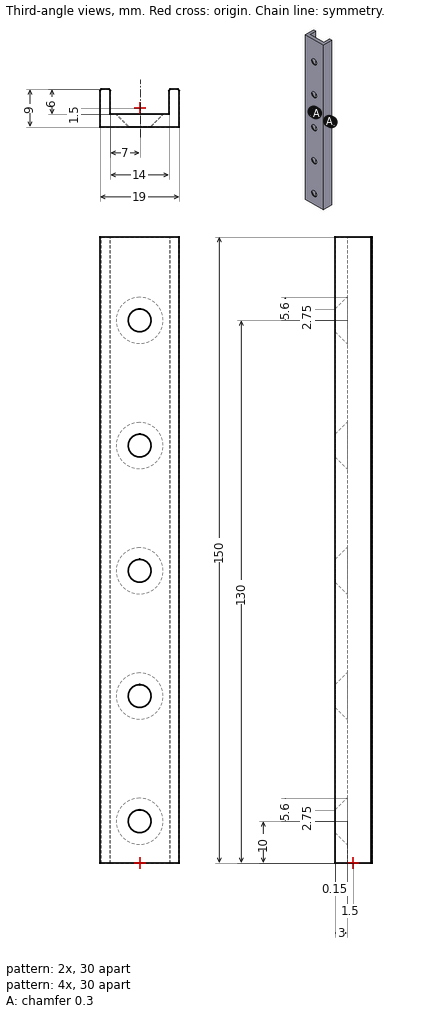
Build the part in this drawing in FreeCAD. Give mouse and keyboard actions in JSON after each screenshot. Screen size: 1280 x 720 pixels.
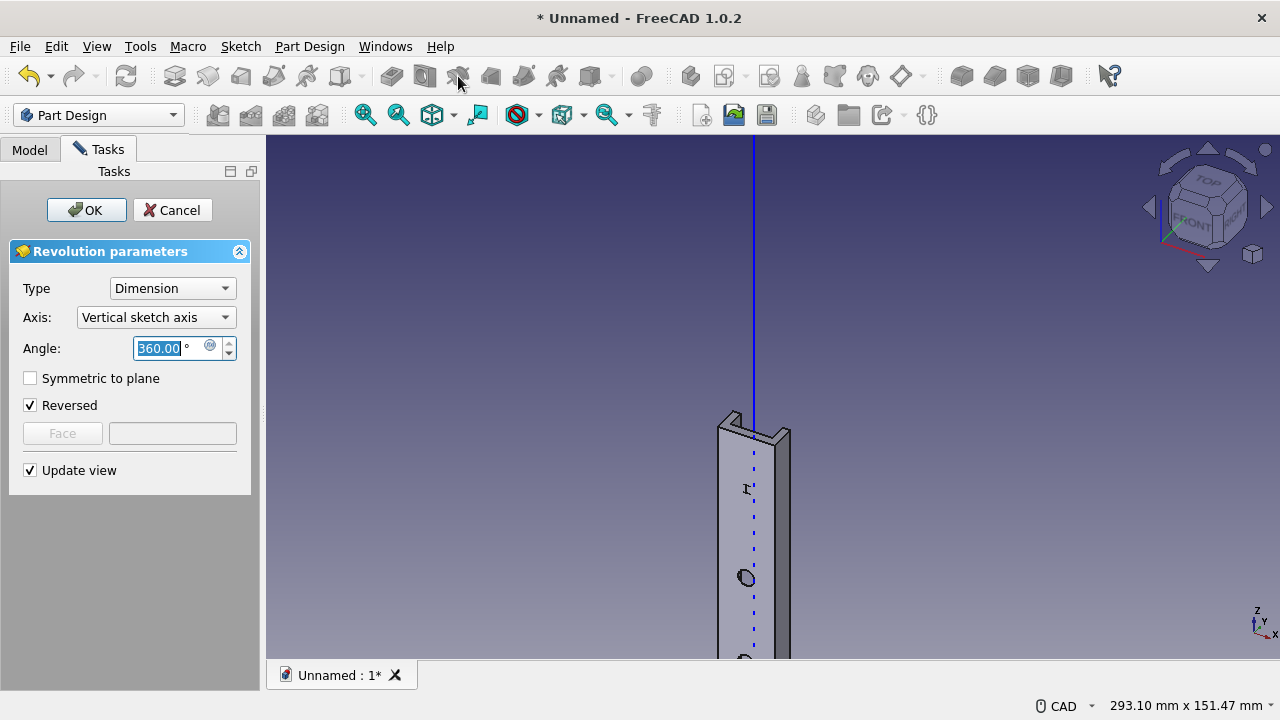
{"action": "left_click", "coordinate": [157, 318]}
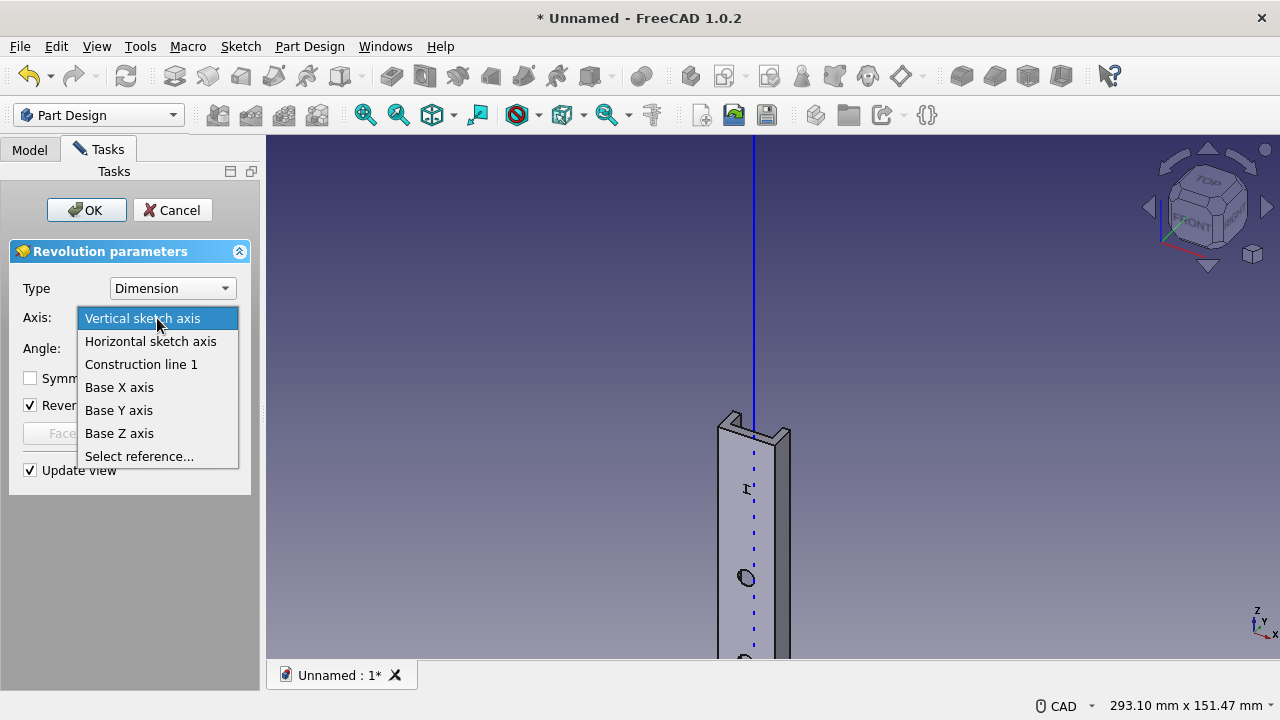
{"action": "left_click", "coordinate": [156, 364]}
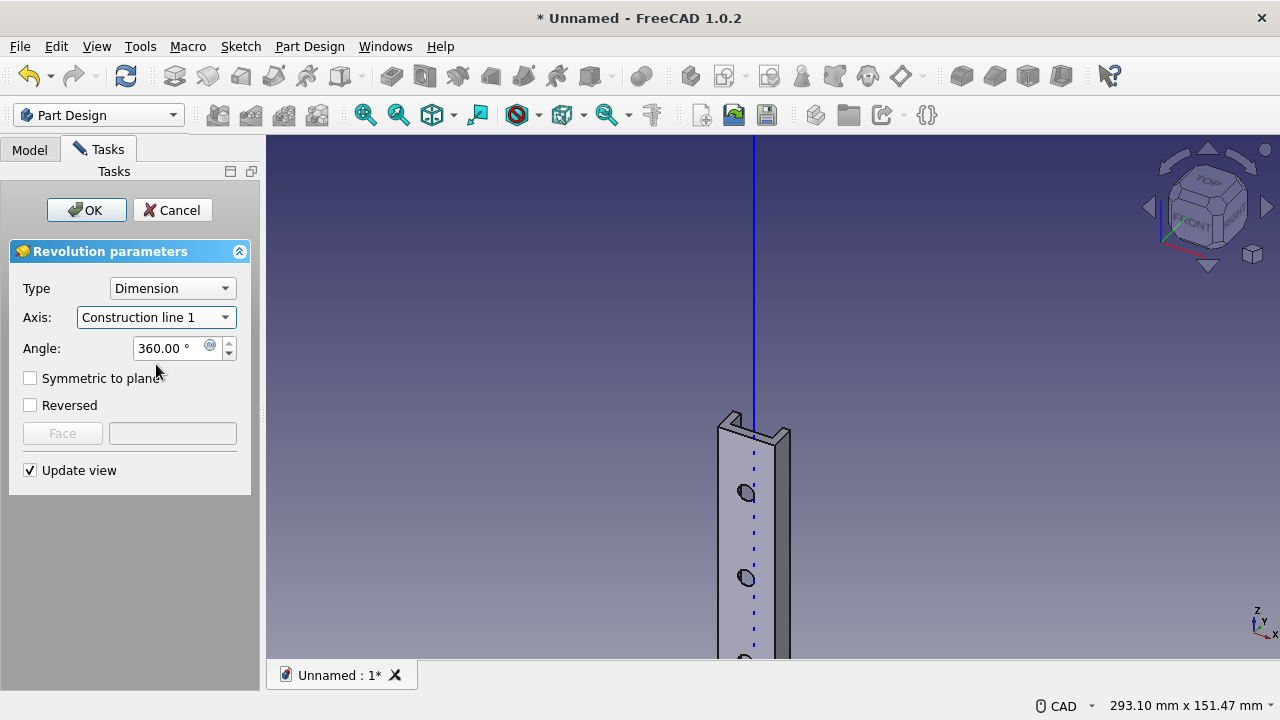
{"action": "left_click", "coordinate": [87, 210]}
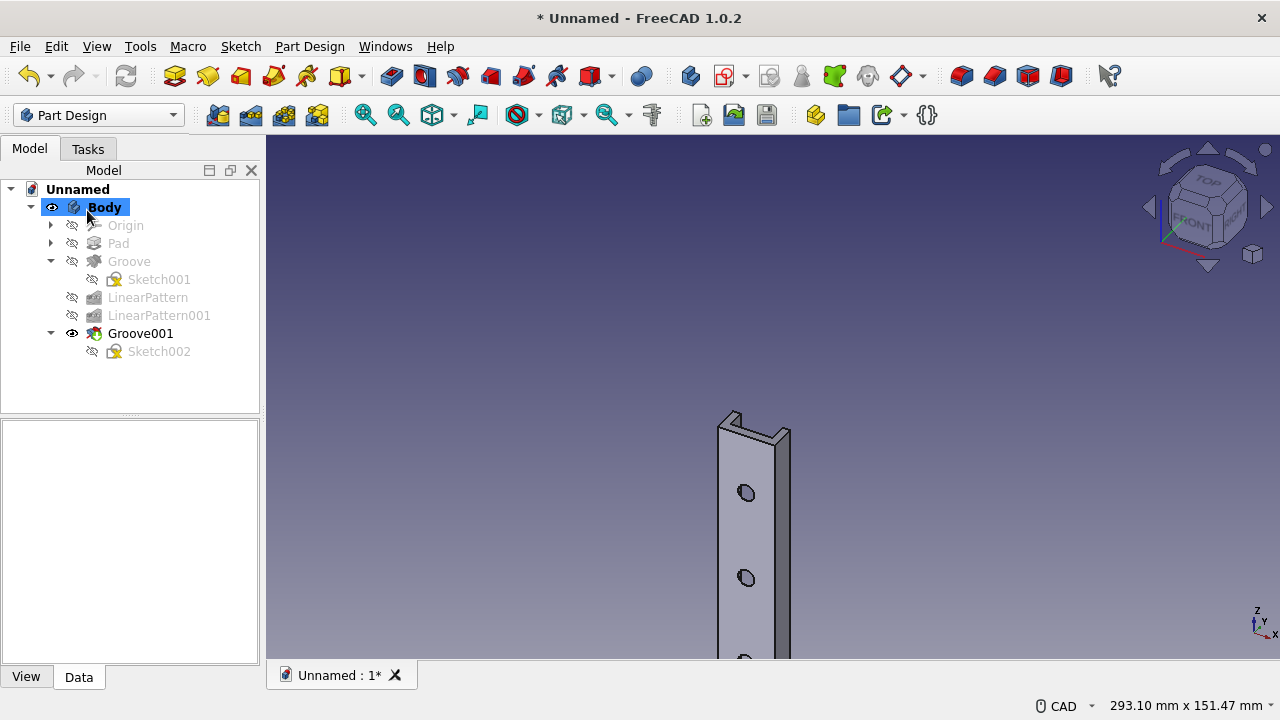
{"action": "key", "text": "v f"}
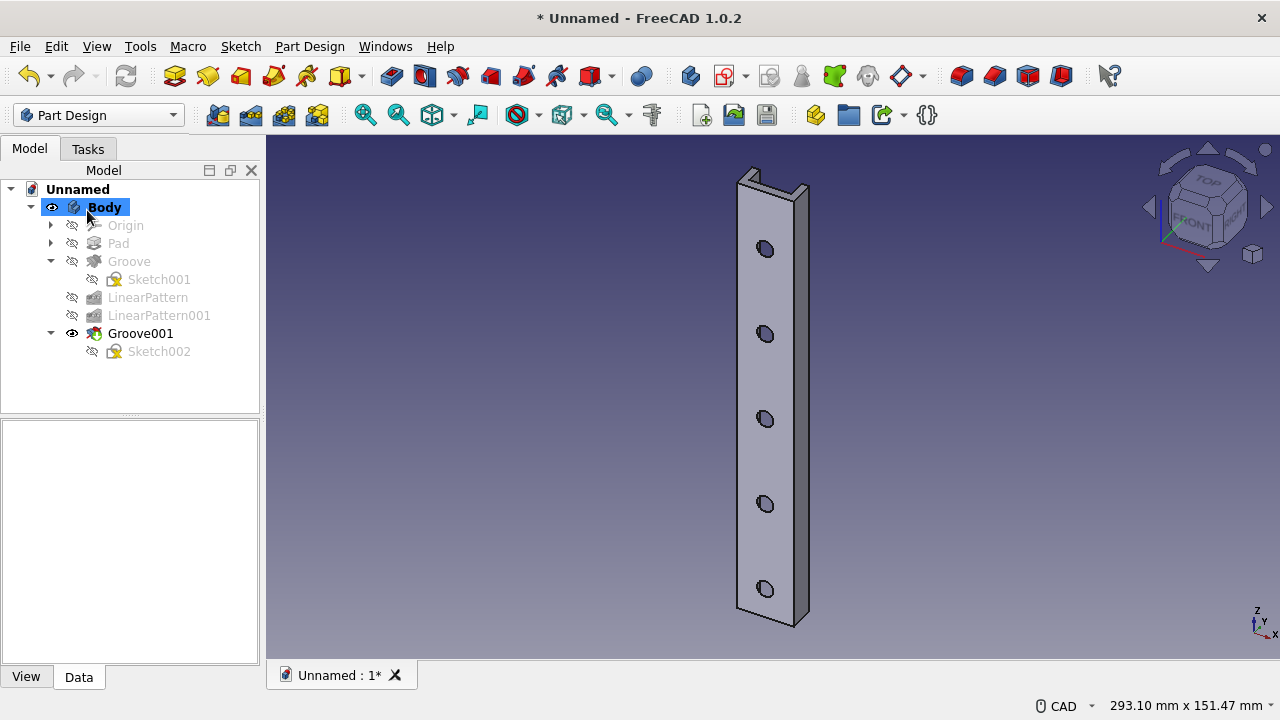
{"action": "key", "text": "0"}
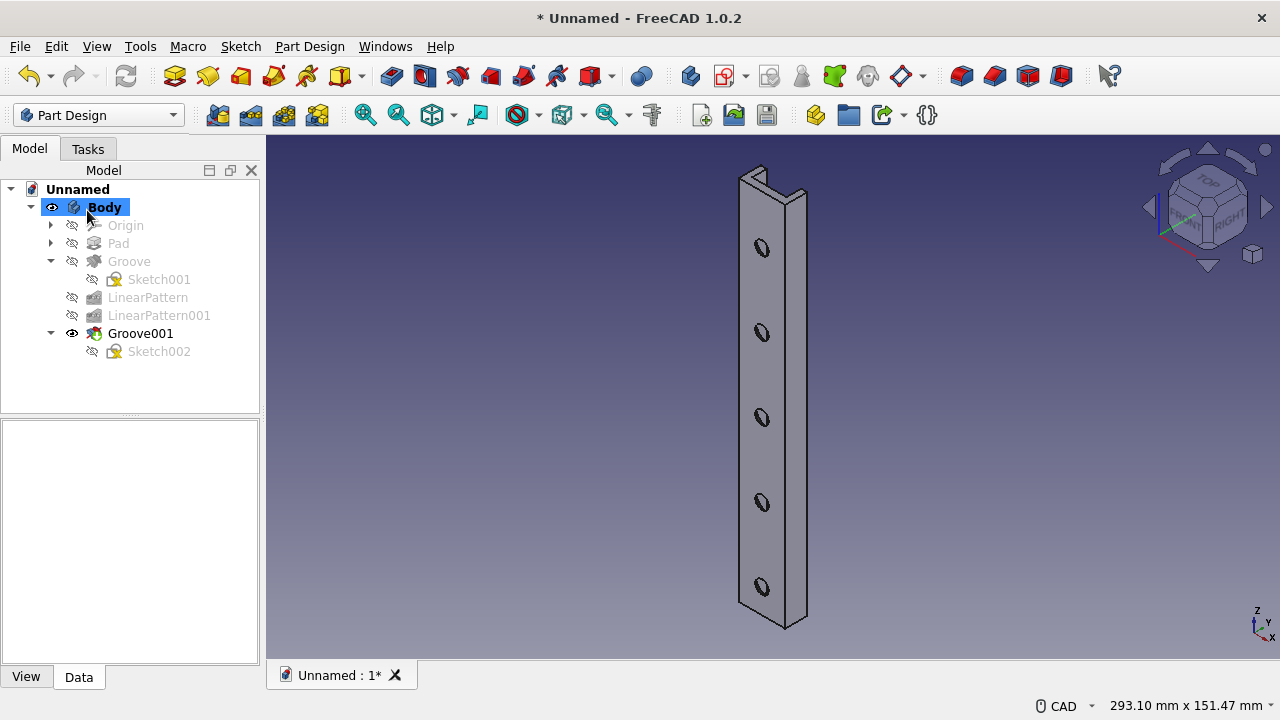
{"action": "key", "text": "2"}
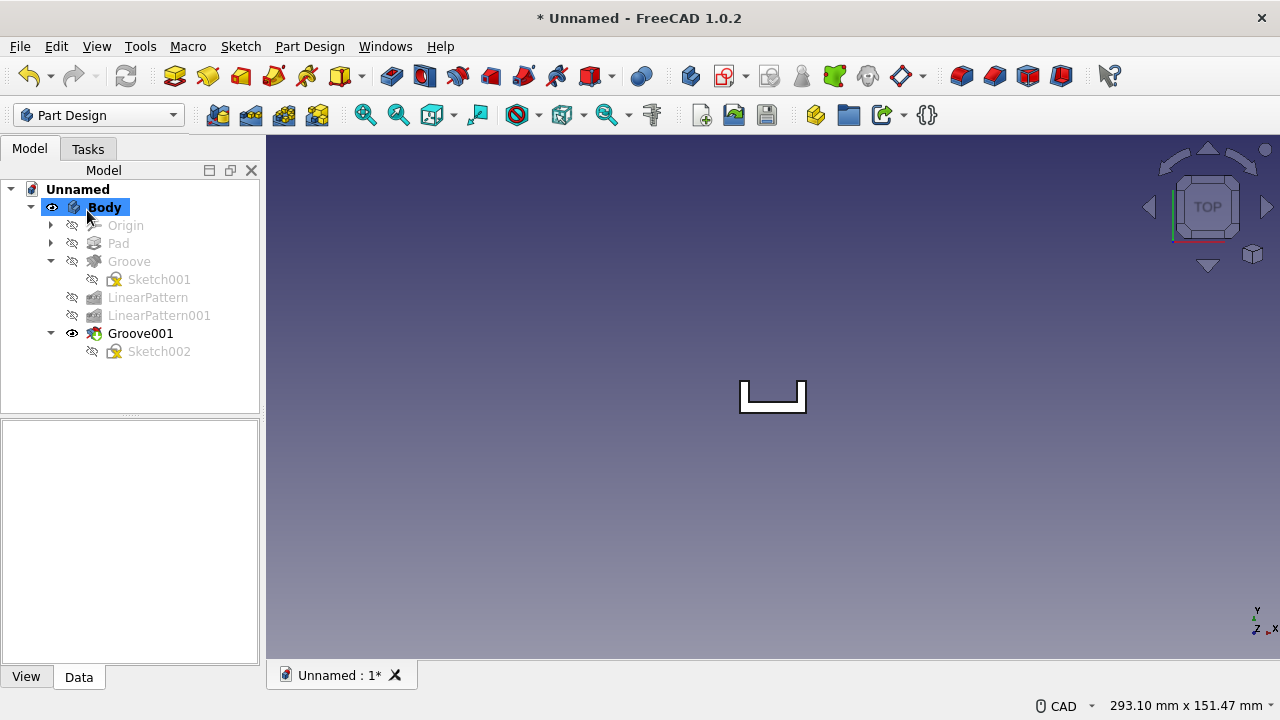
{"action": "left_click", "coordinate": [366, 116]}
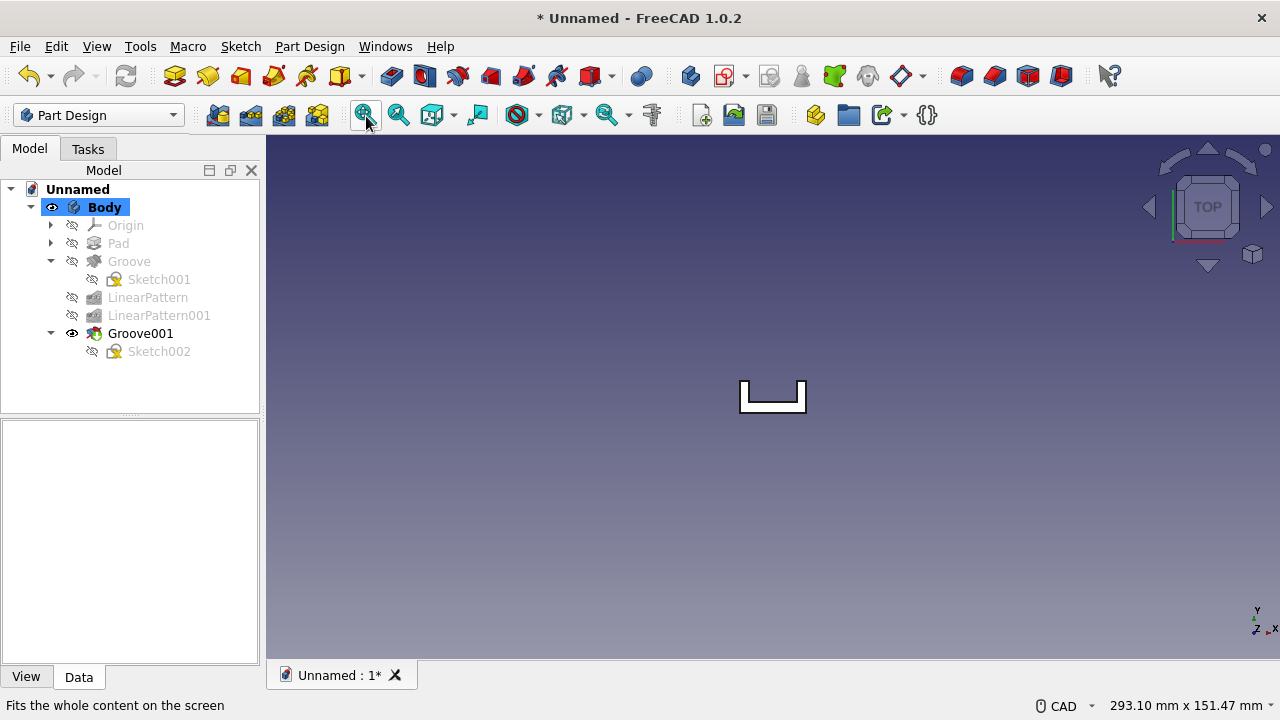
{"action": "key", "text": "1"}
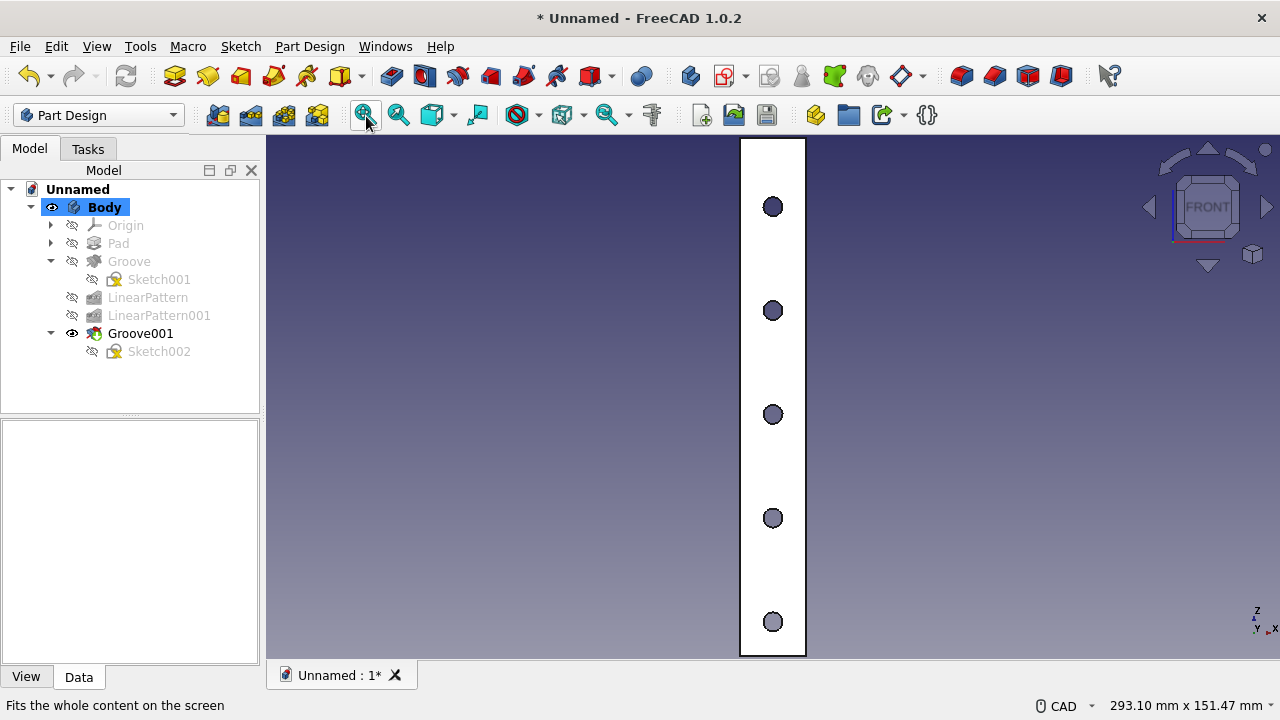
{"action": "key", "text": "3"}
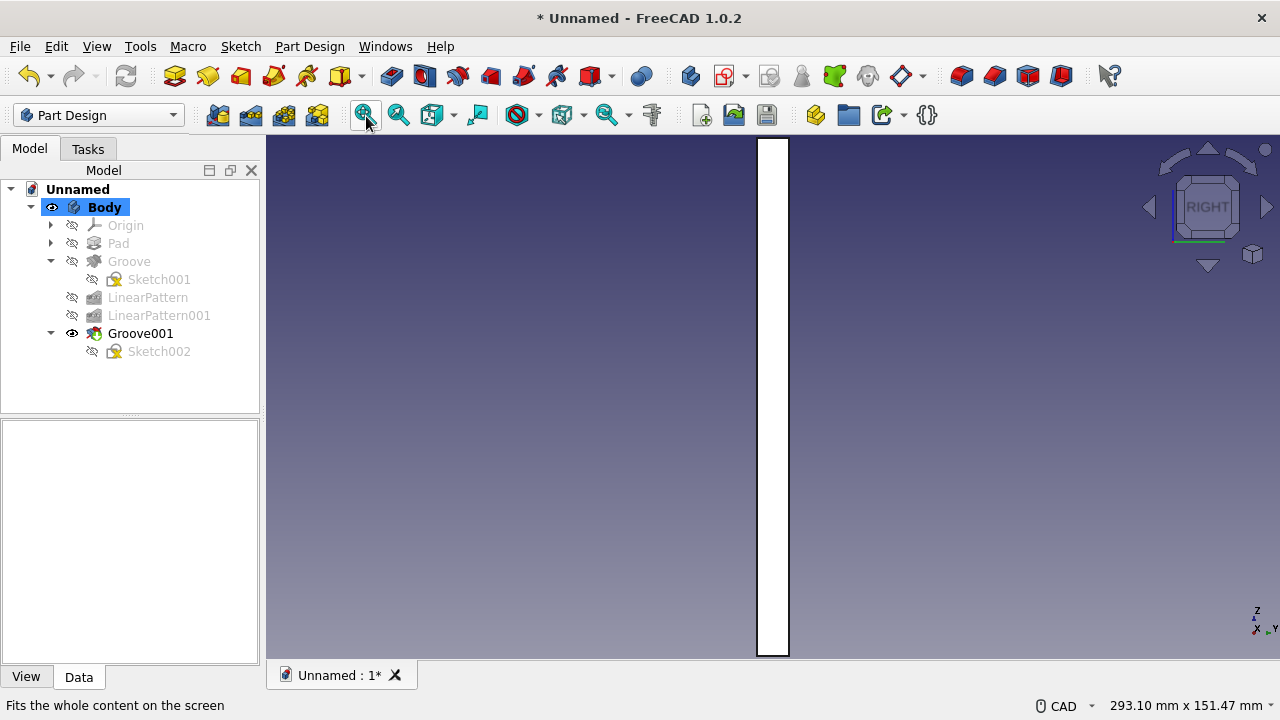
{"action": "left_click", "coordinate": [789, 396]}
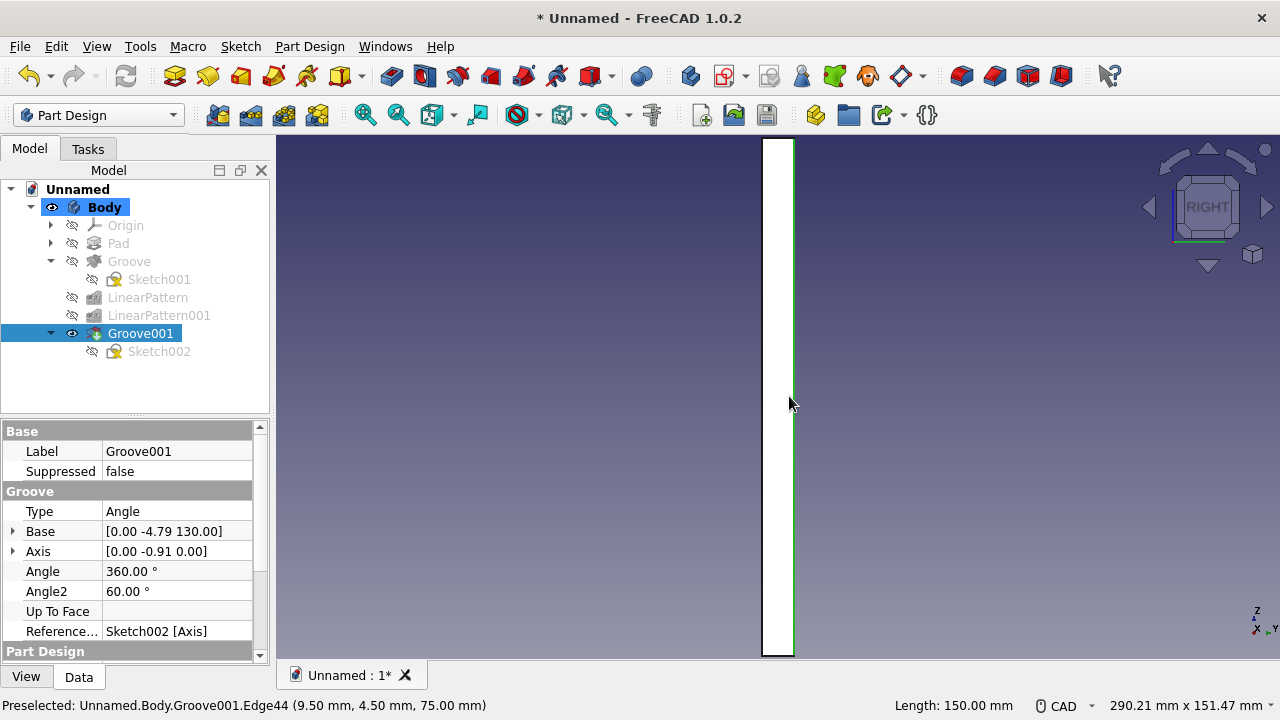
{"action": "key", "text": "5"}